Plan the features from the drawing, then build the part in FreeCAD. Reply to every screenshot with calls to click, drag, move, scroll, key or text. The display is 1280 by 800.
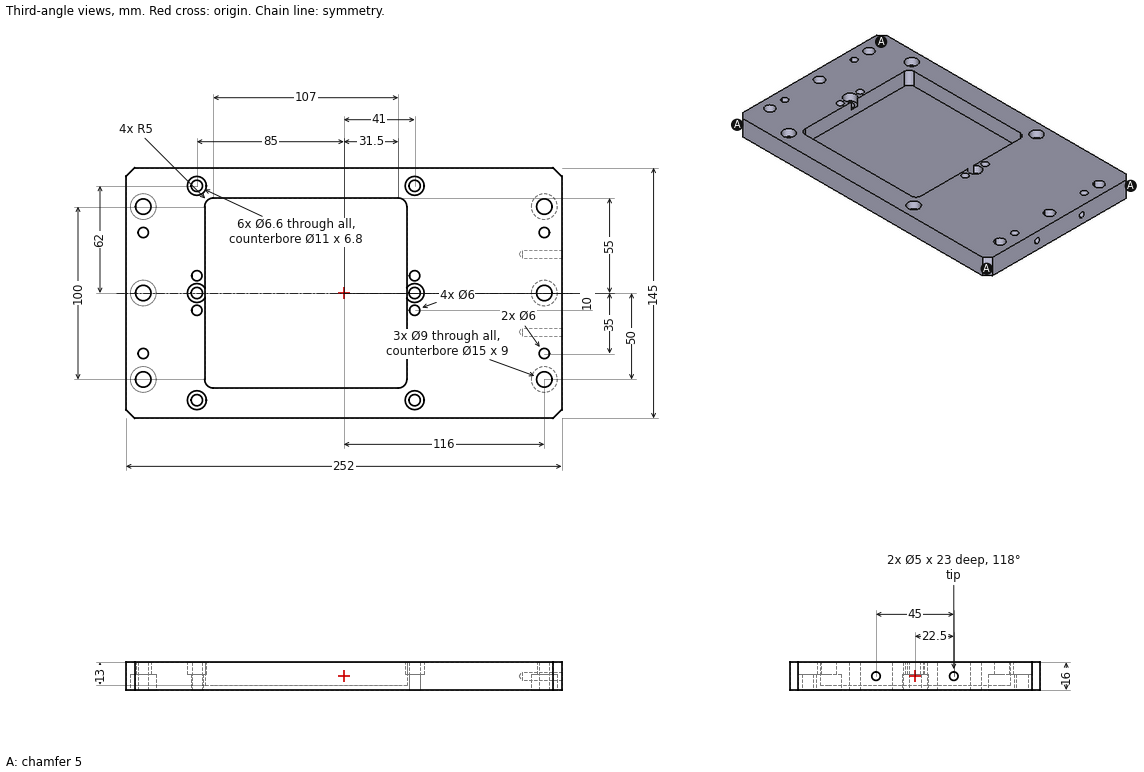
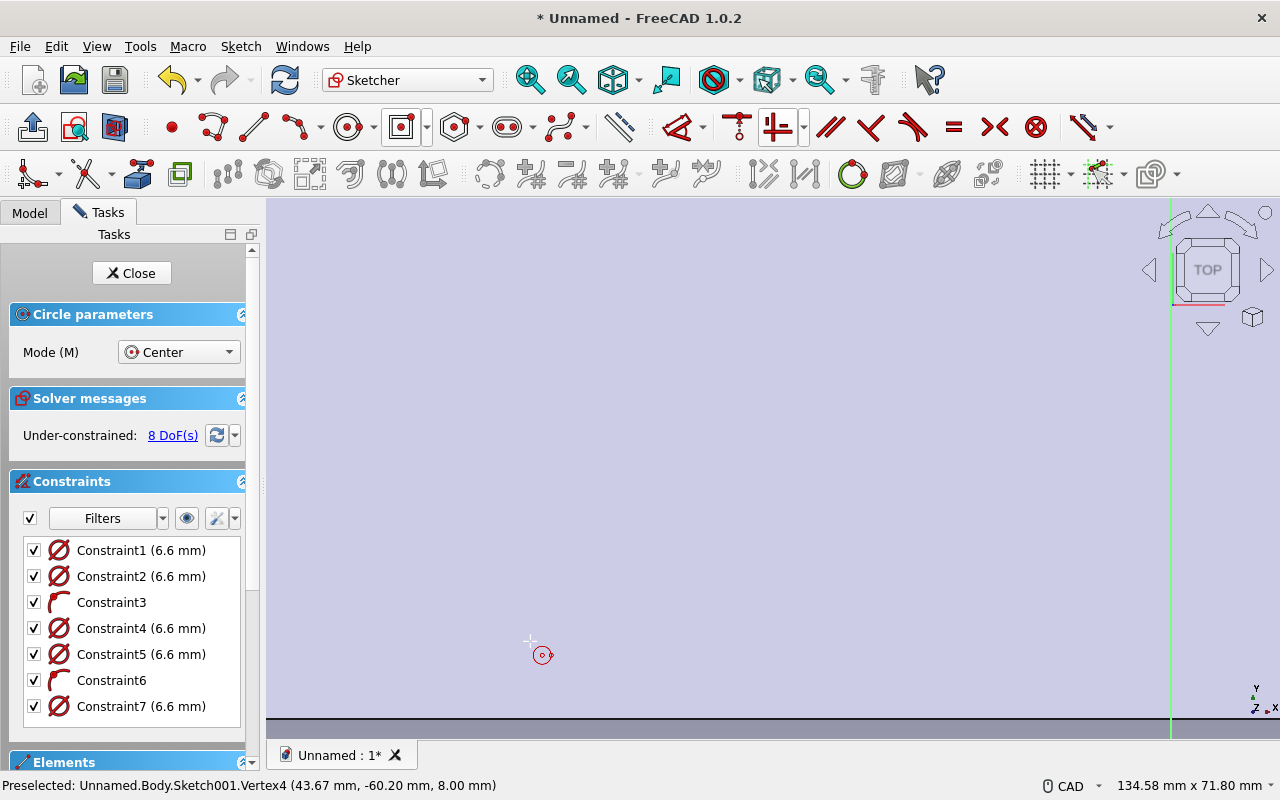
click(531, 640)
move(548, 622)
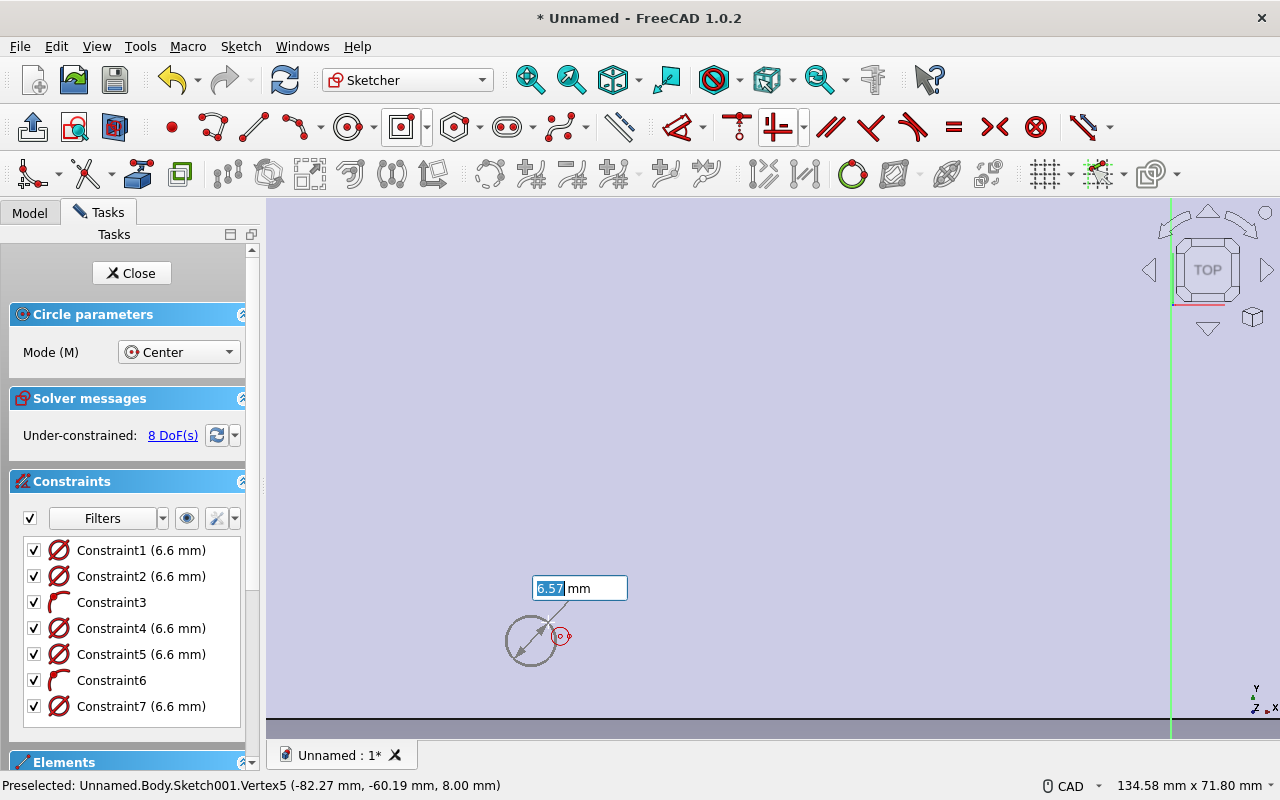
text(6.6)
key(Return)
key(Escape)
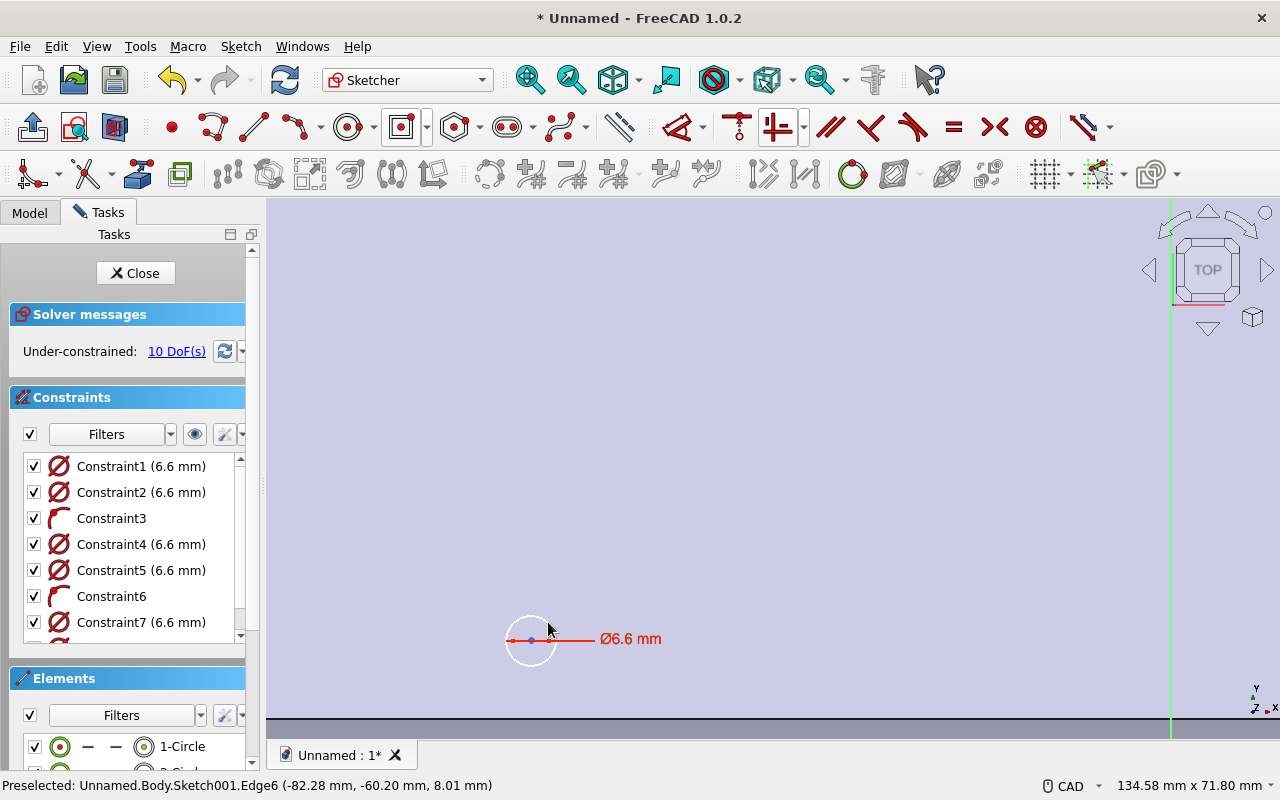
scroll(529, 641, down, 5)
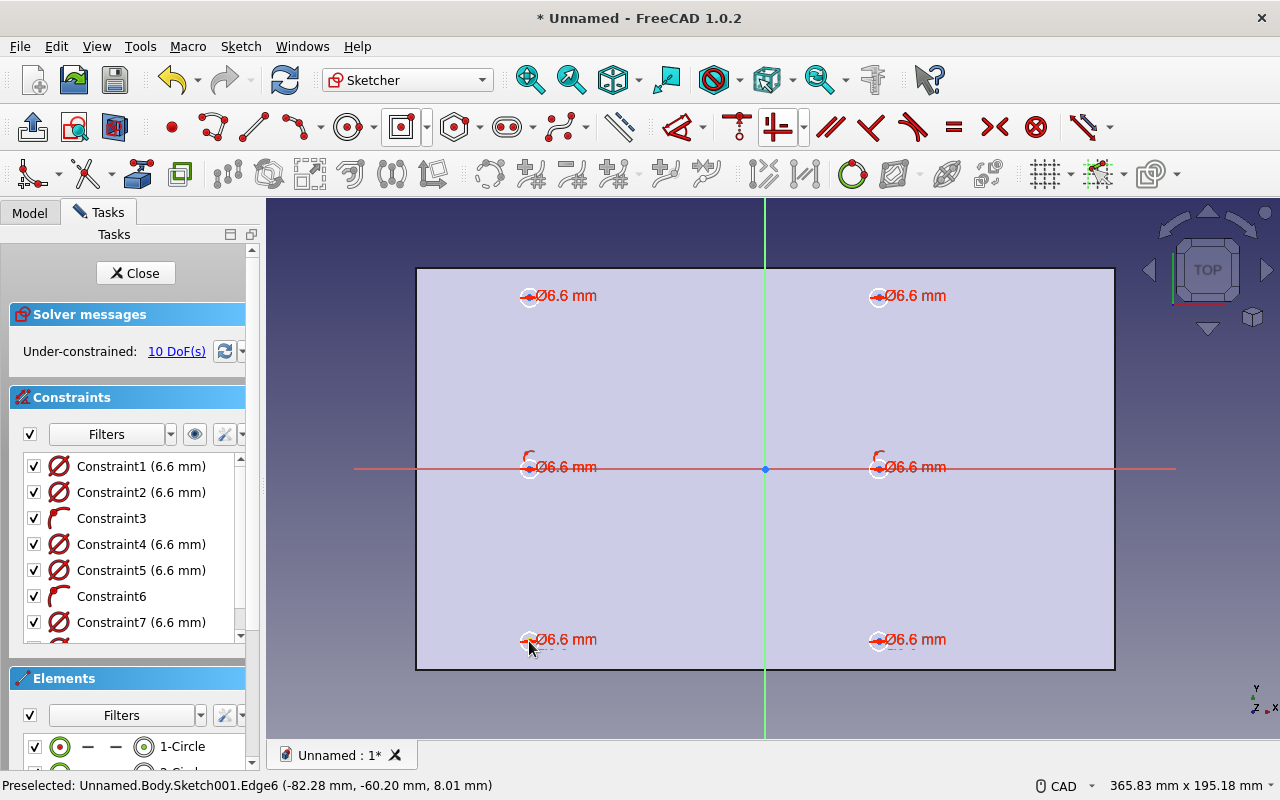
click(879, 298)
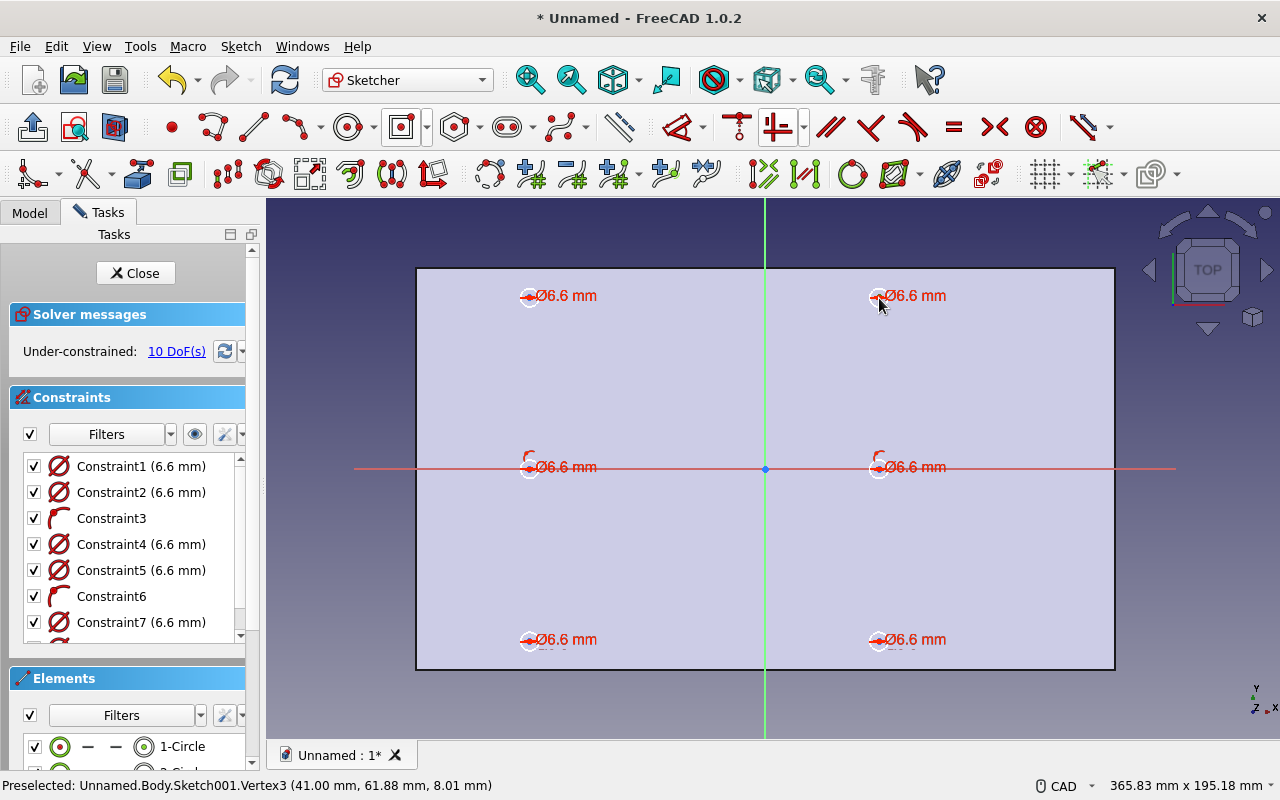
click(879, 642)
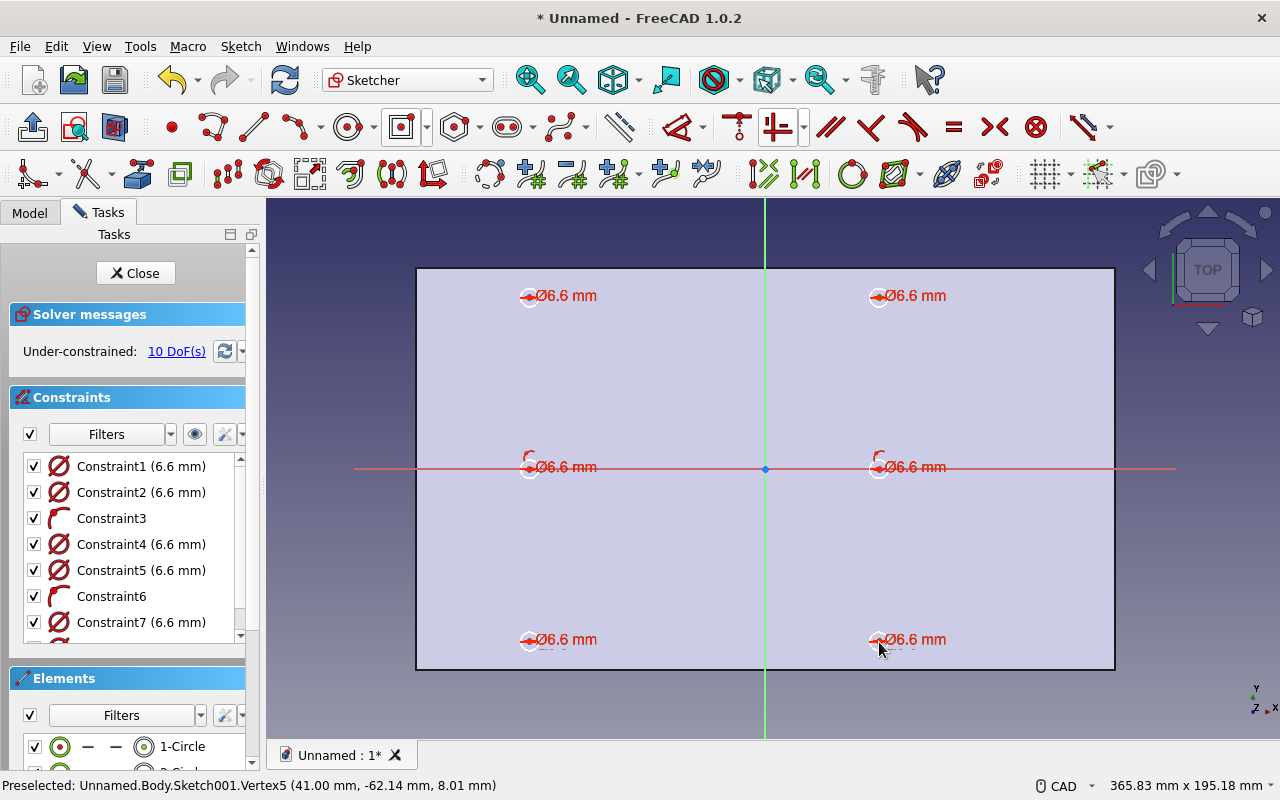
click(353, 469)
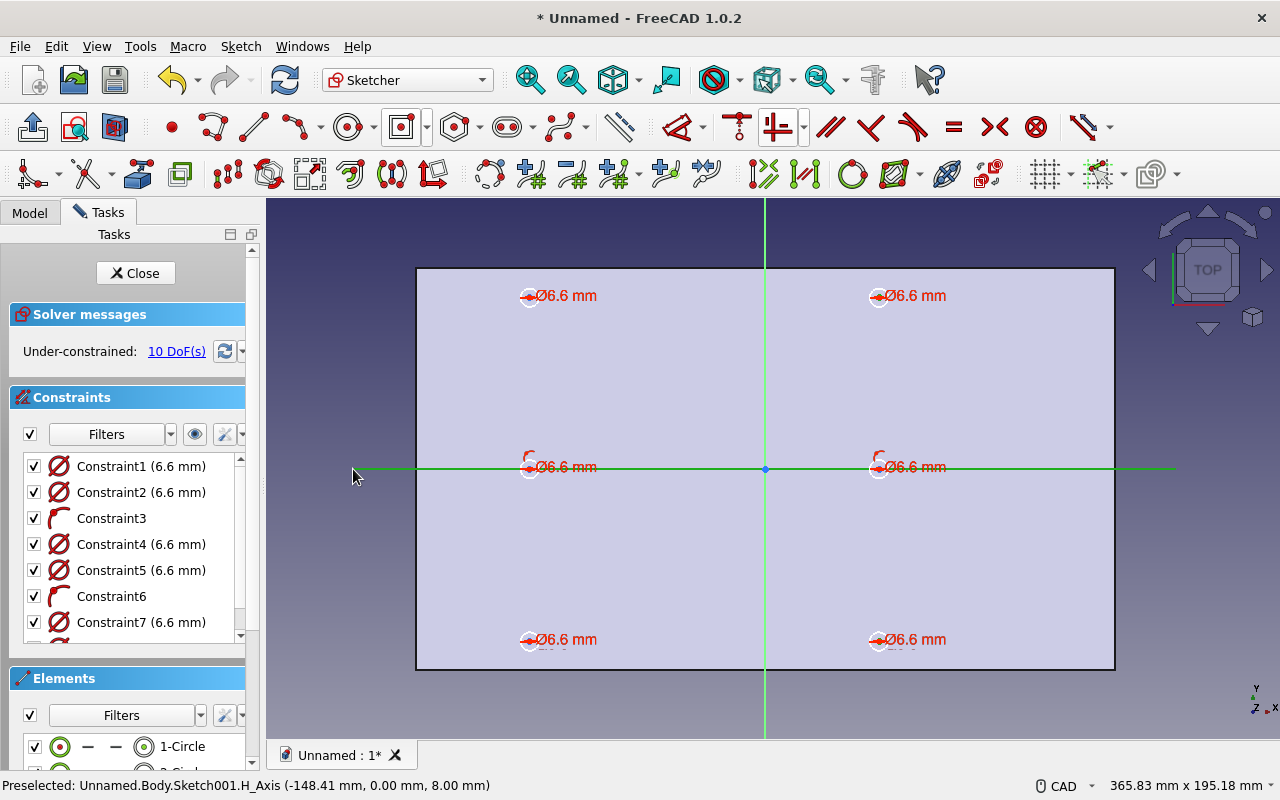
key(s)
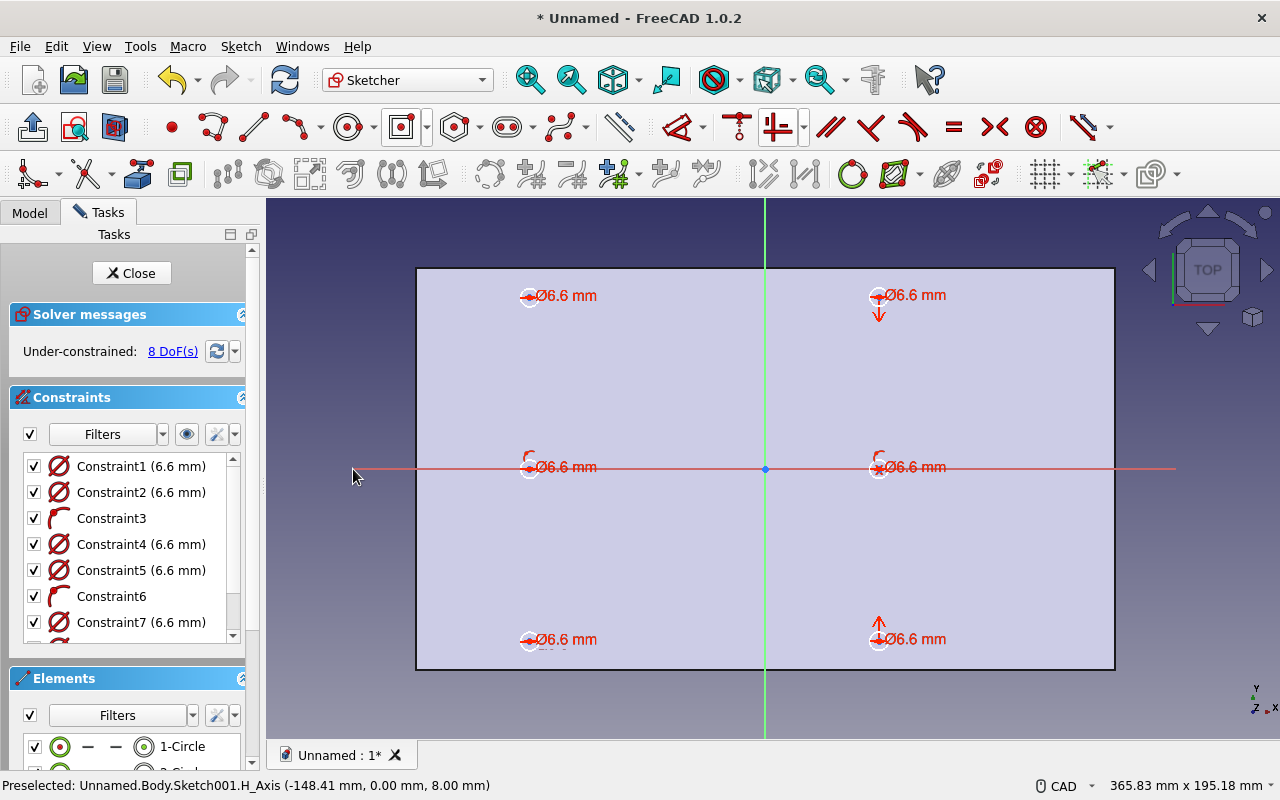
click(530, 298)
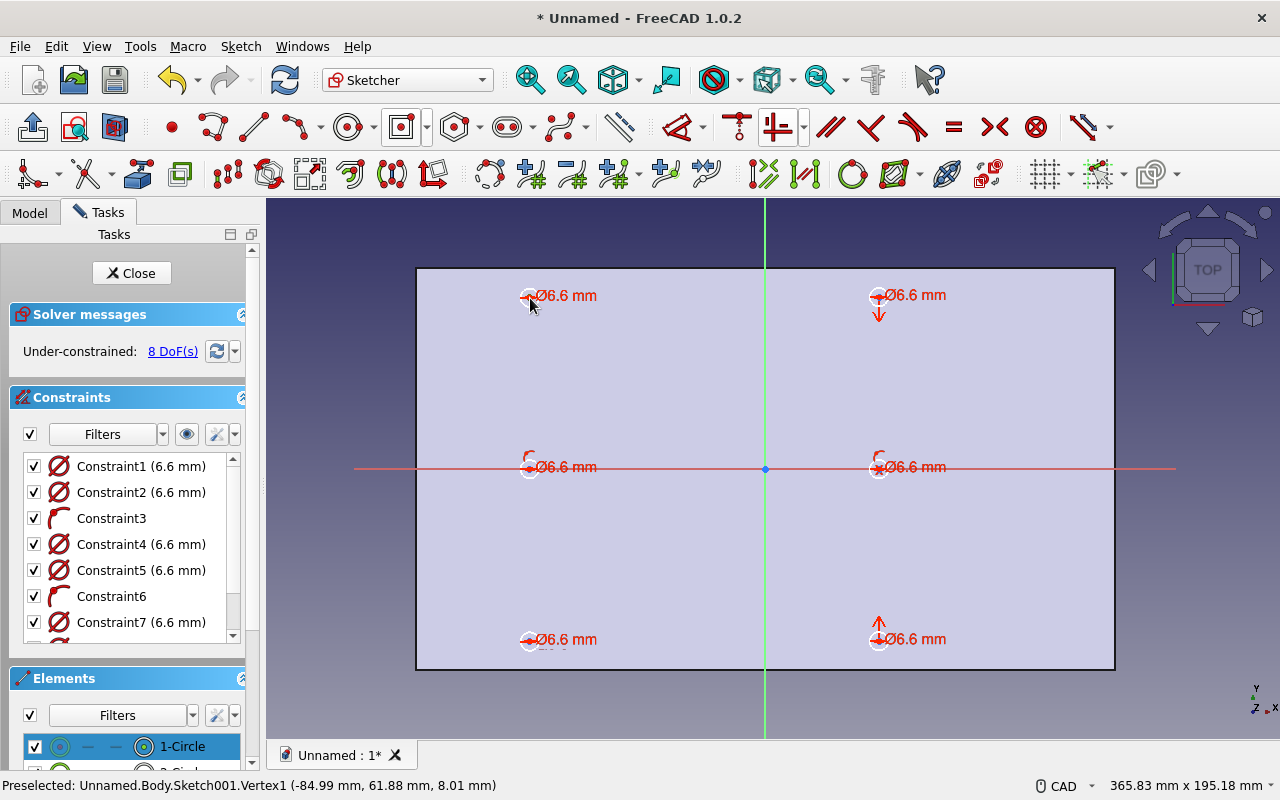
click(530, 642)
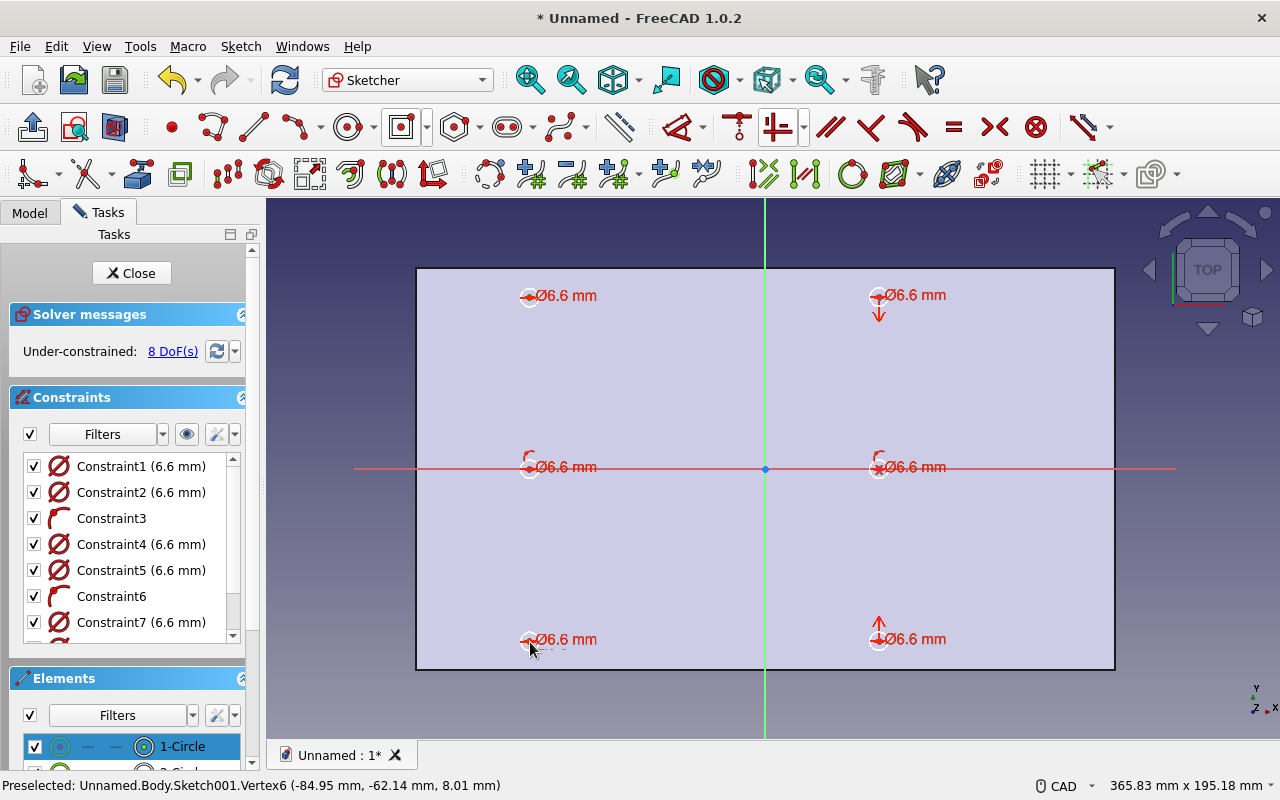
click(353, 469)